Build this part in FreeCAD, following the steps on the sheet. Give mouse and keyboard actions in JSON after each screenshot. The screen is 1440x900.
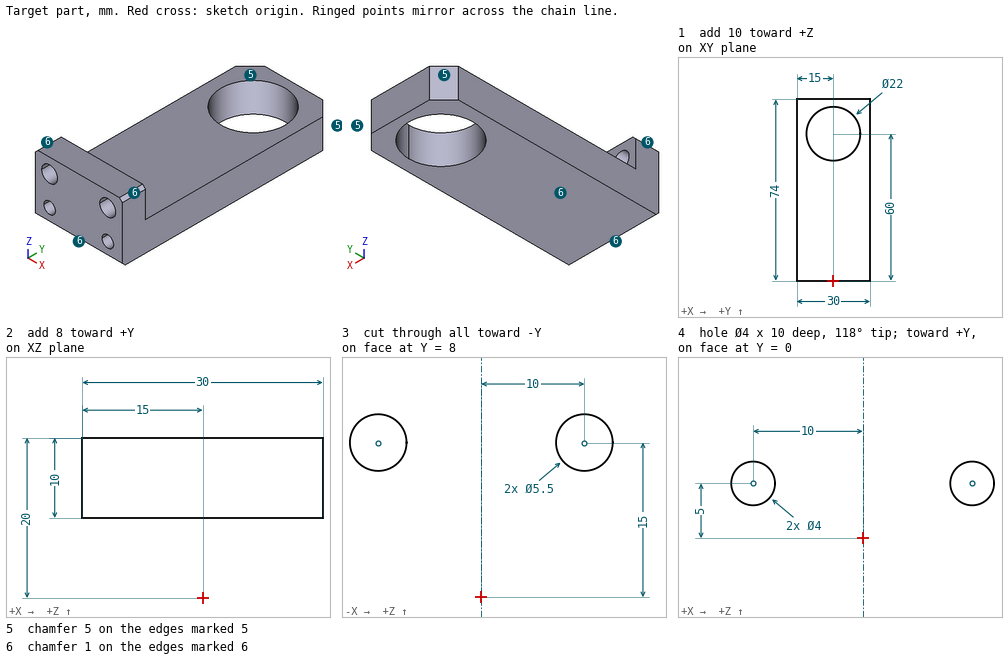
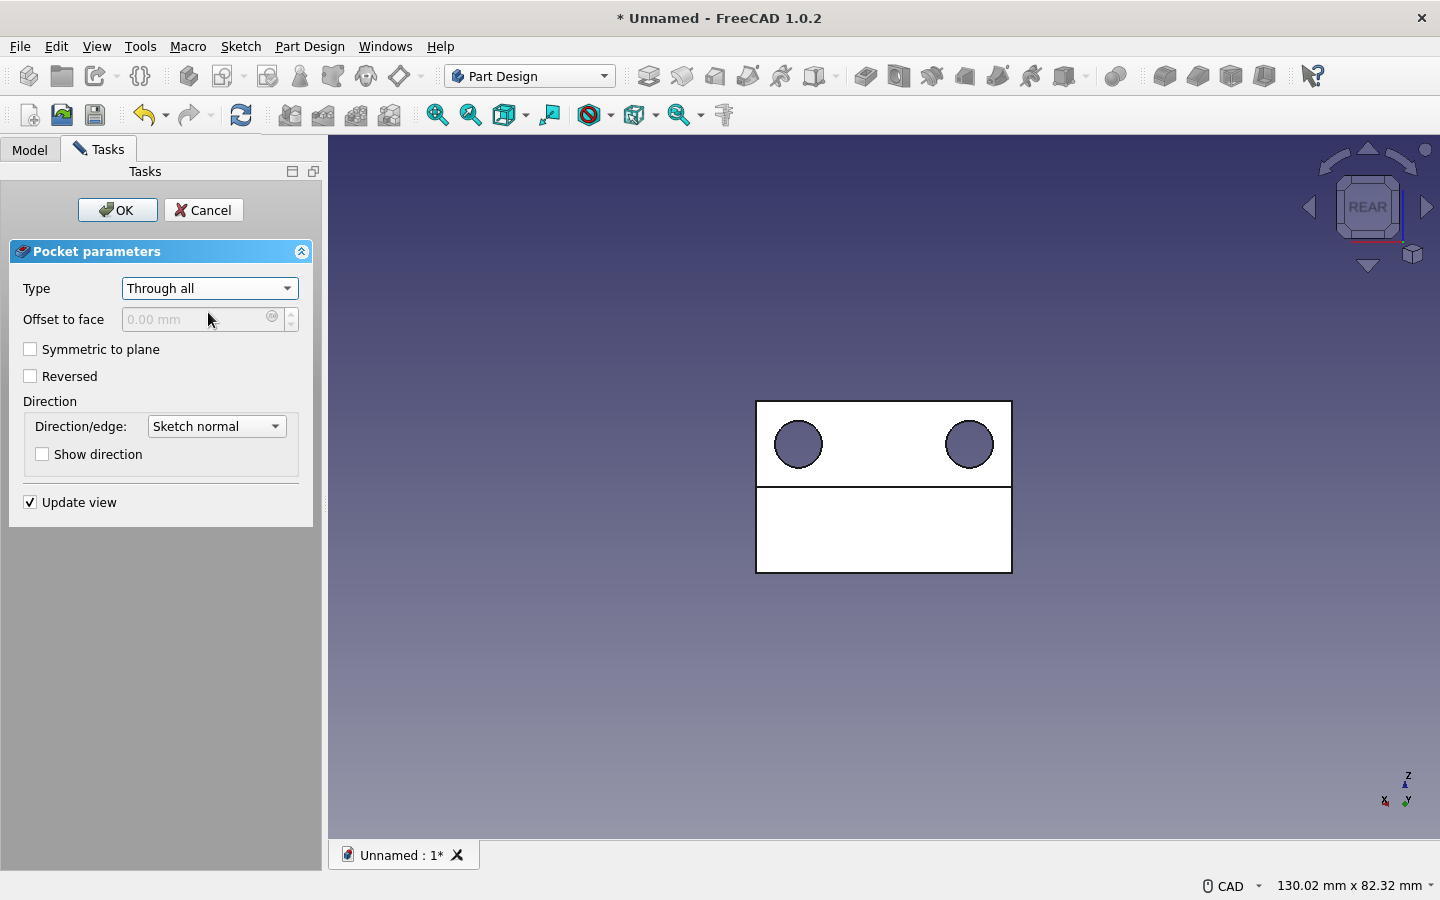
{"action": "left_click", "coordinate": [118, 210]}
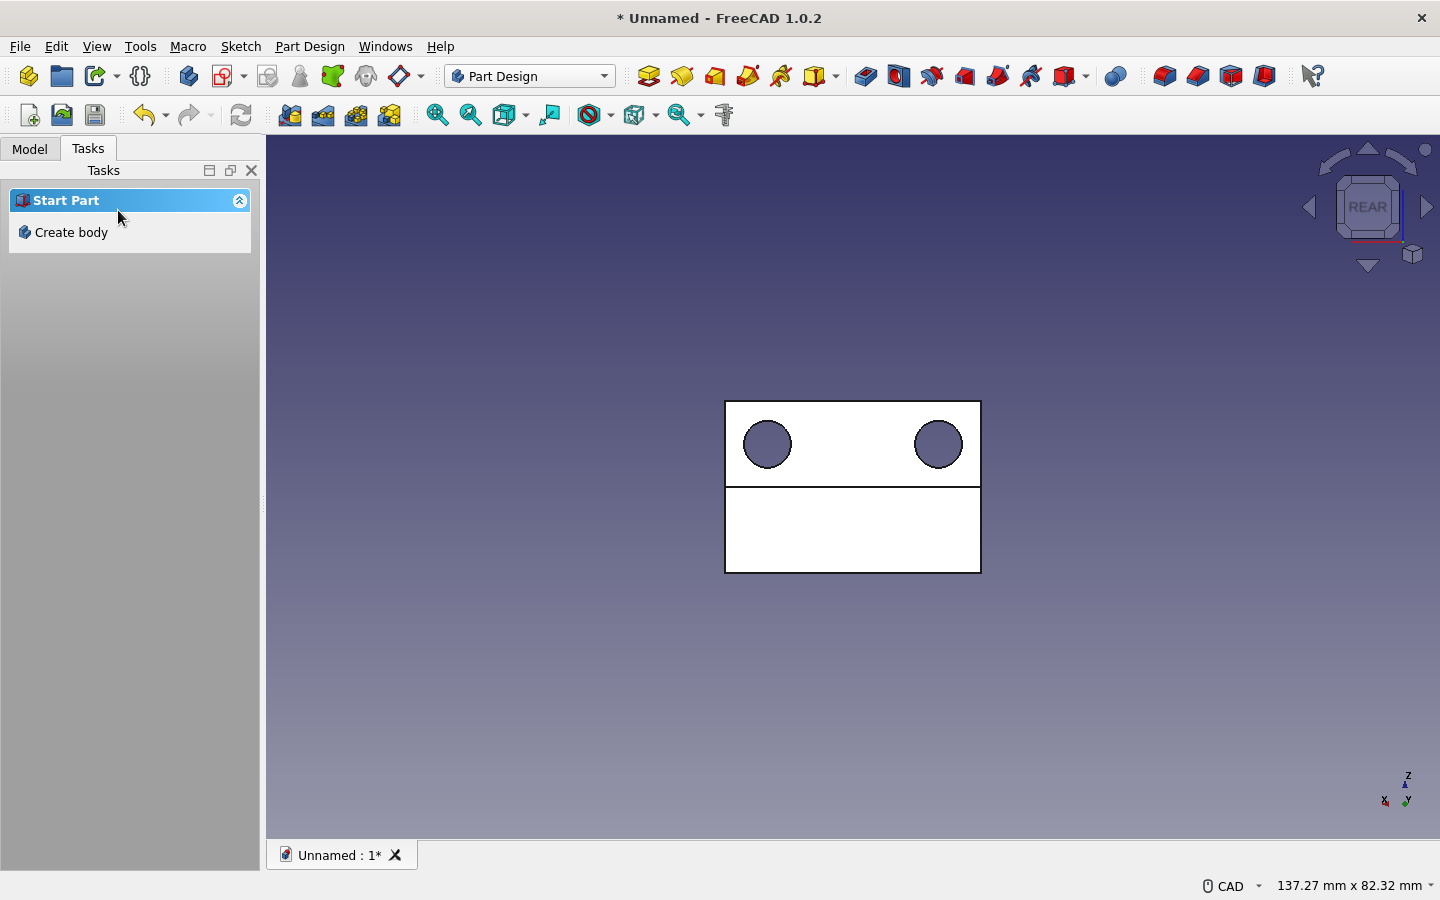
{"action": "left_click", "coordinate": [438, 116]}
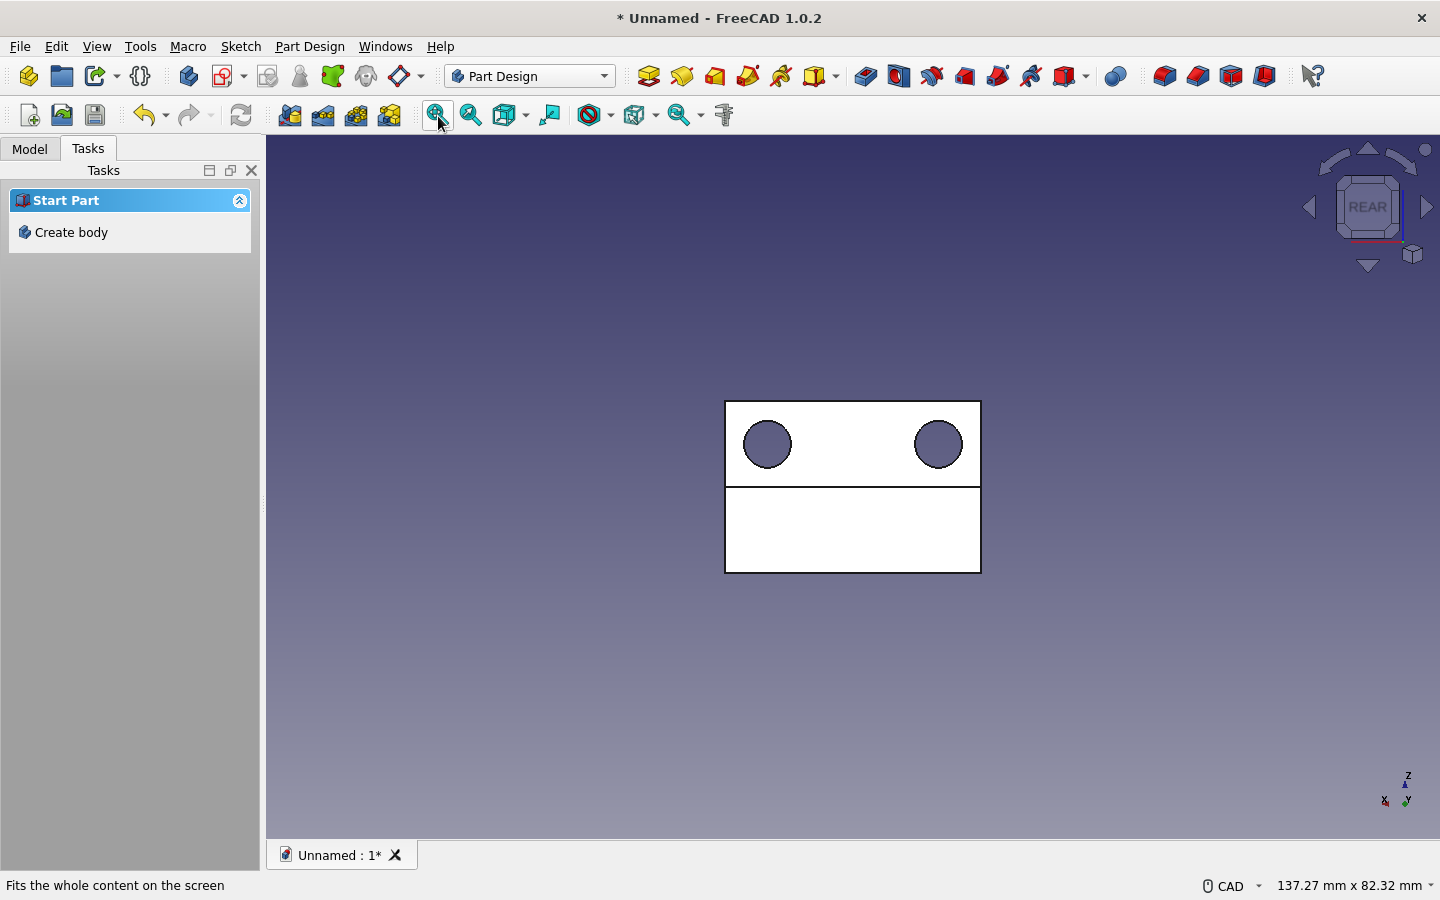
{"action": "key", "text": "0"}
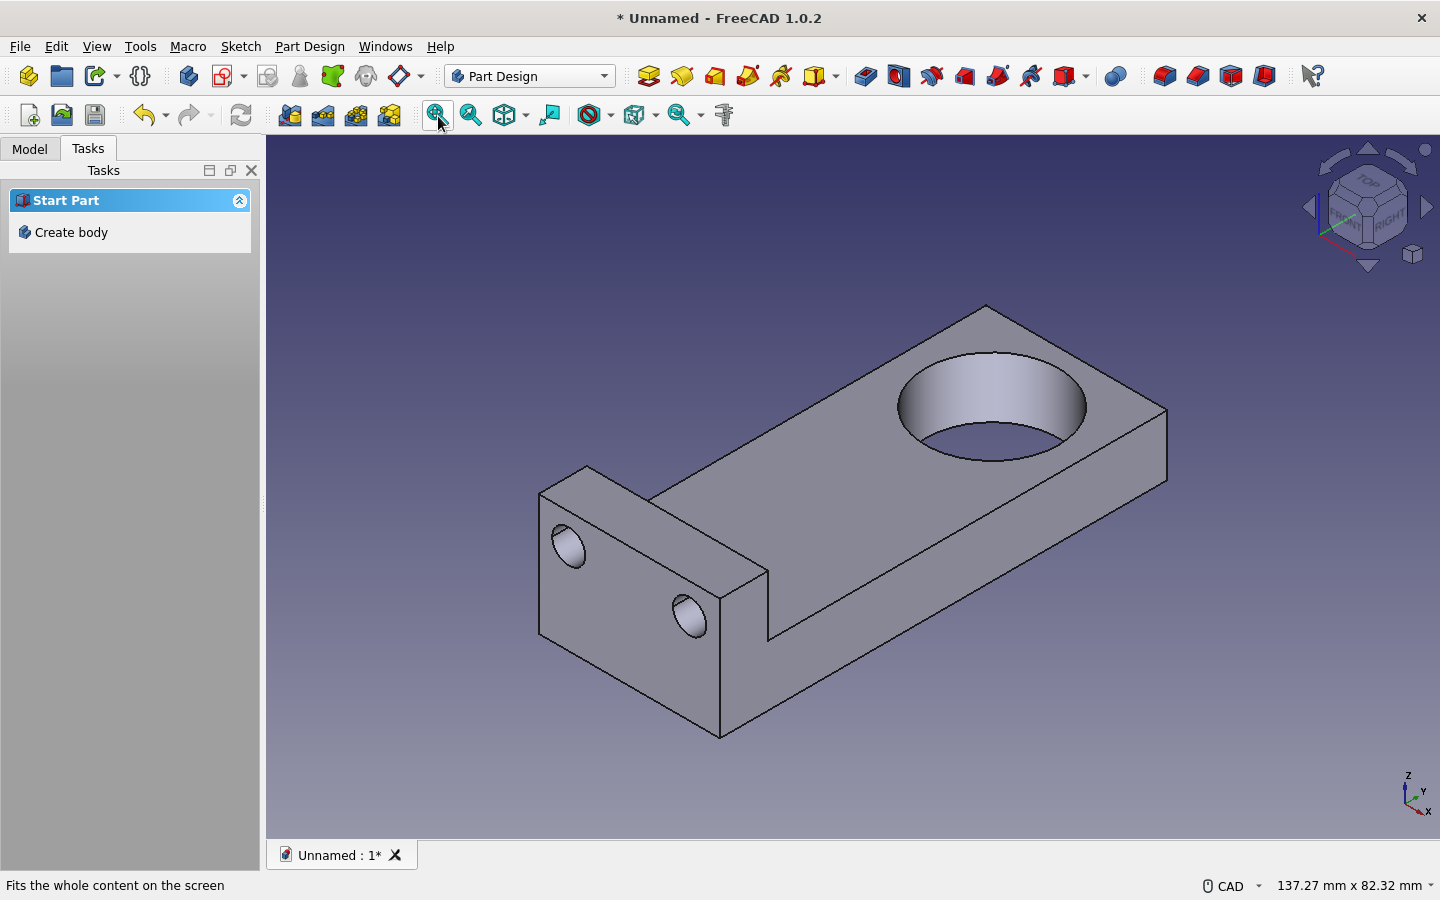
{"action": "left_click", "coordinate": [629, 615]}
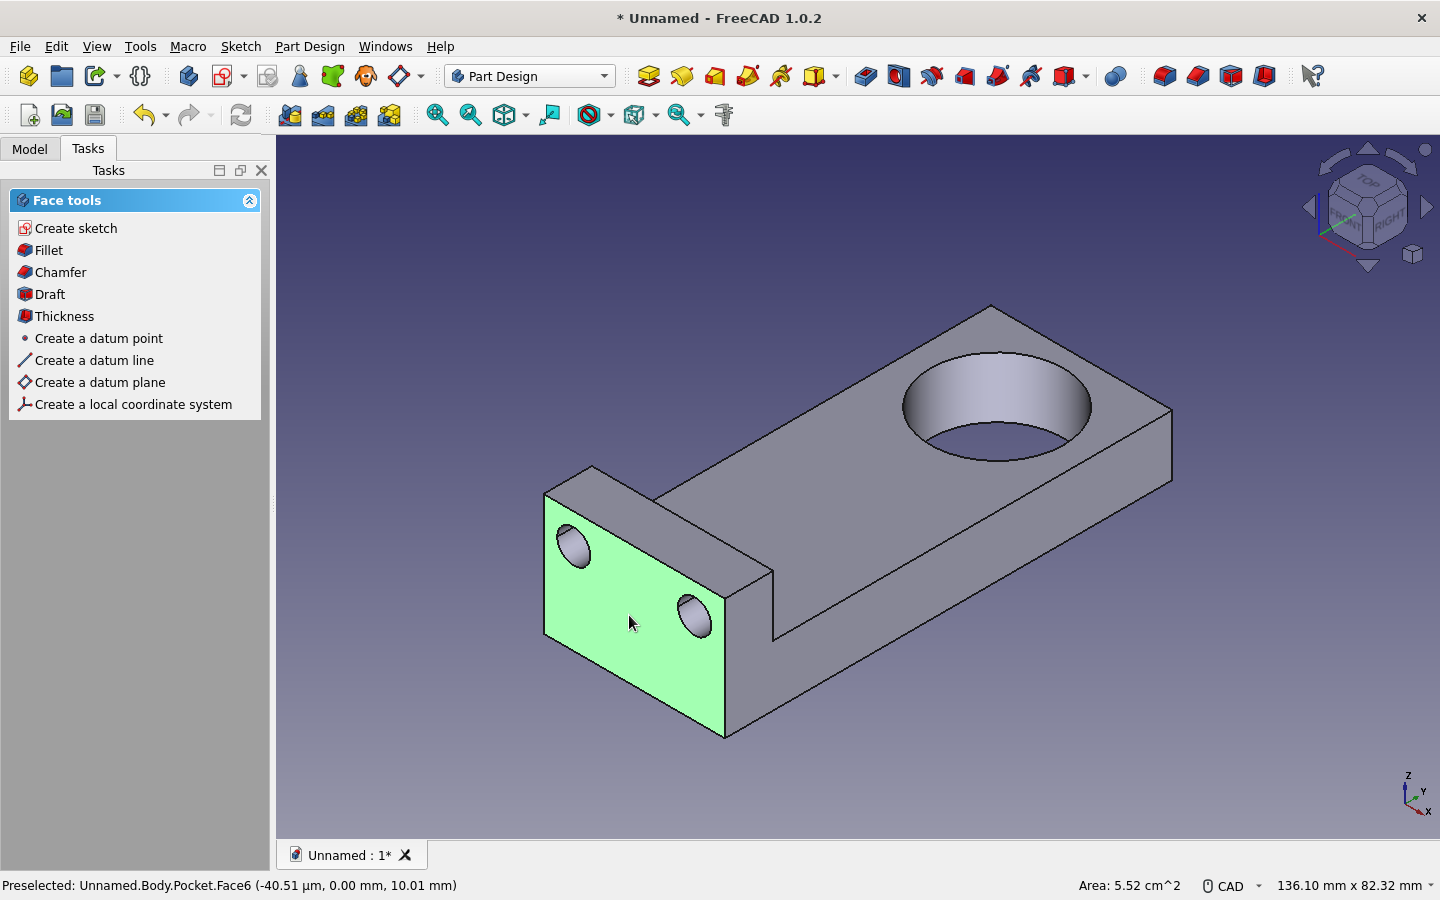
{"action": "left_click", "coordinate": [222, 76]}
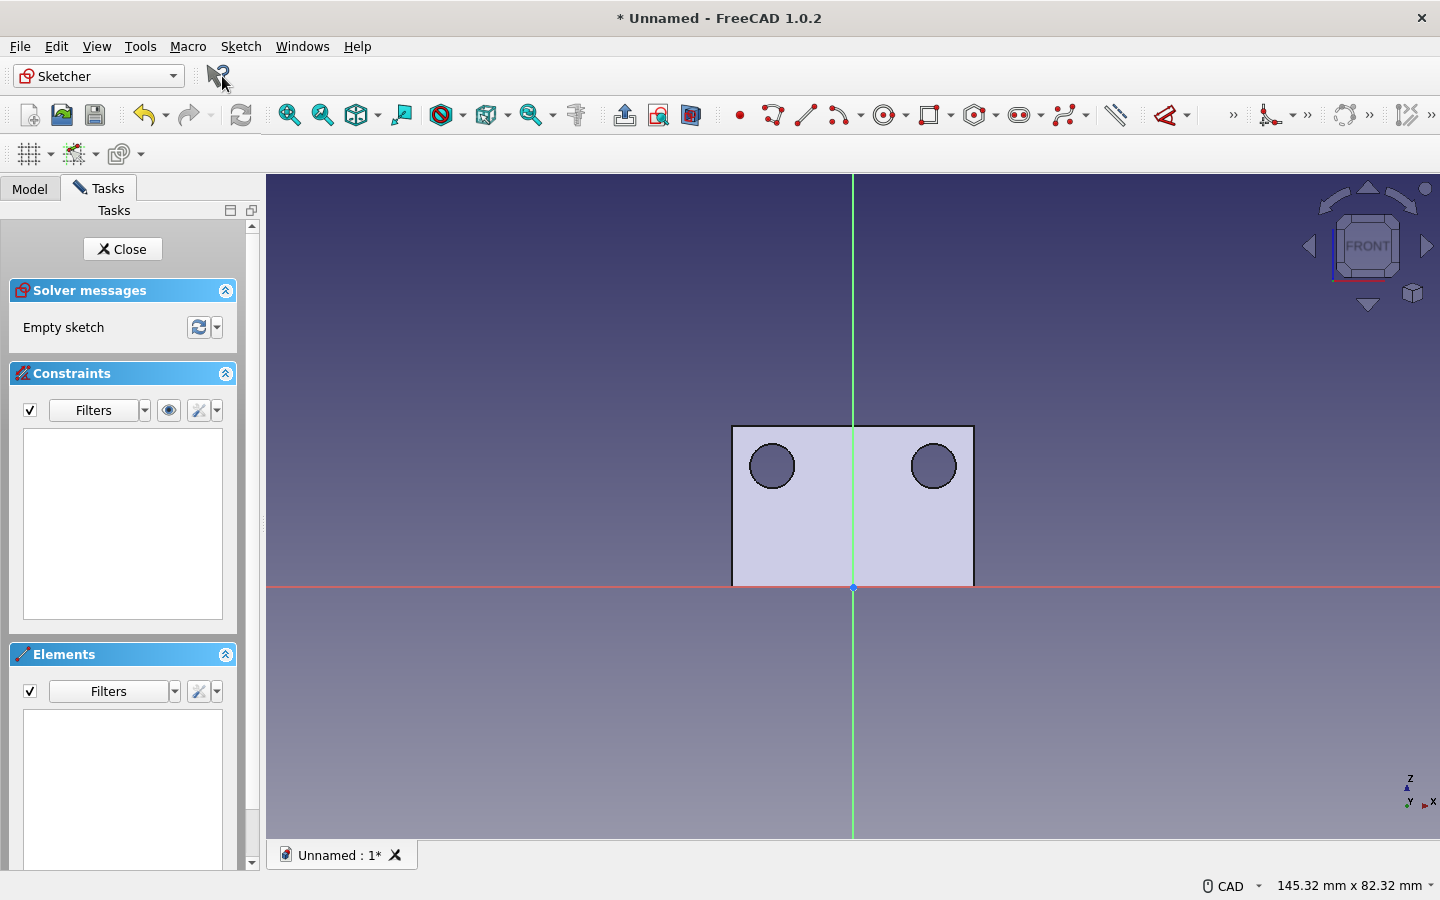
{"action": "scroll", "coordinate": [883, 582], "scroll_direction": "up", "scroll_amount": 6}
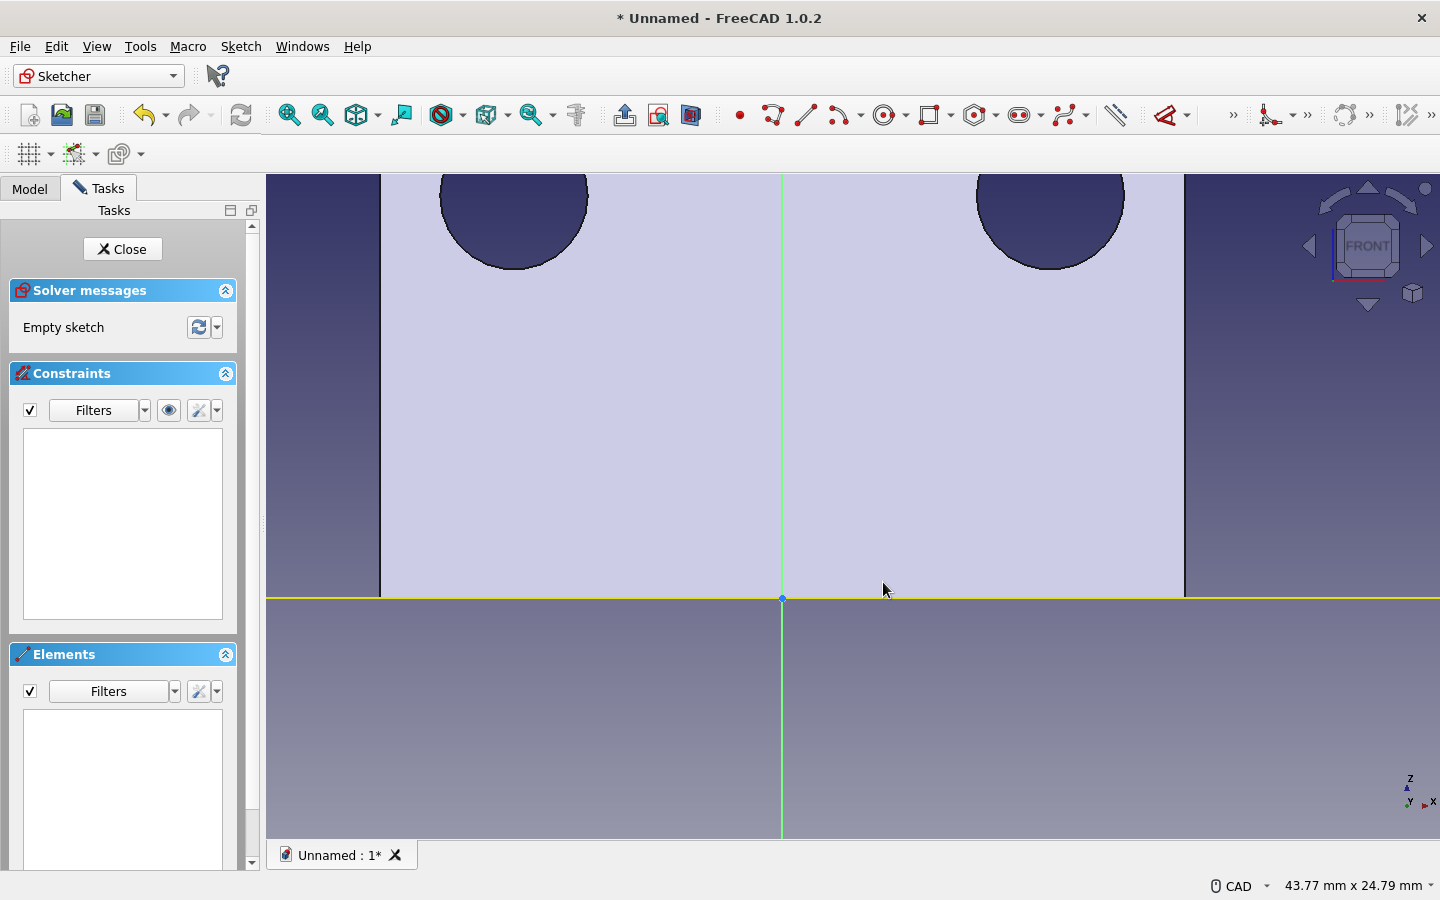
{"action": "left_click", "coordinate": [884, 116]}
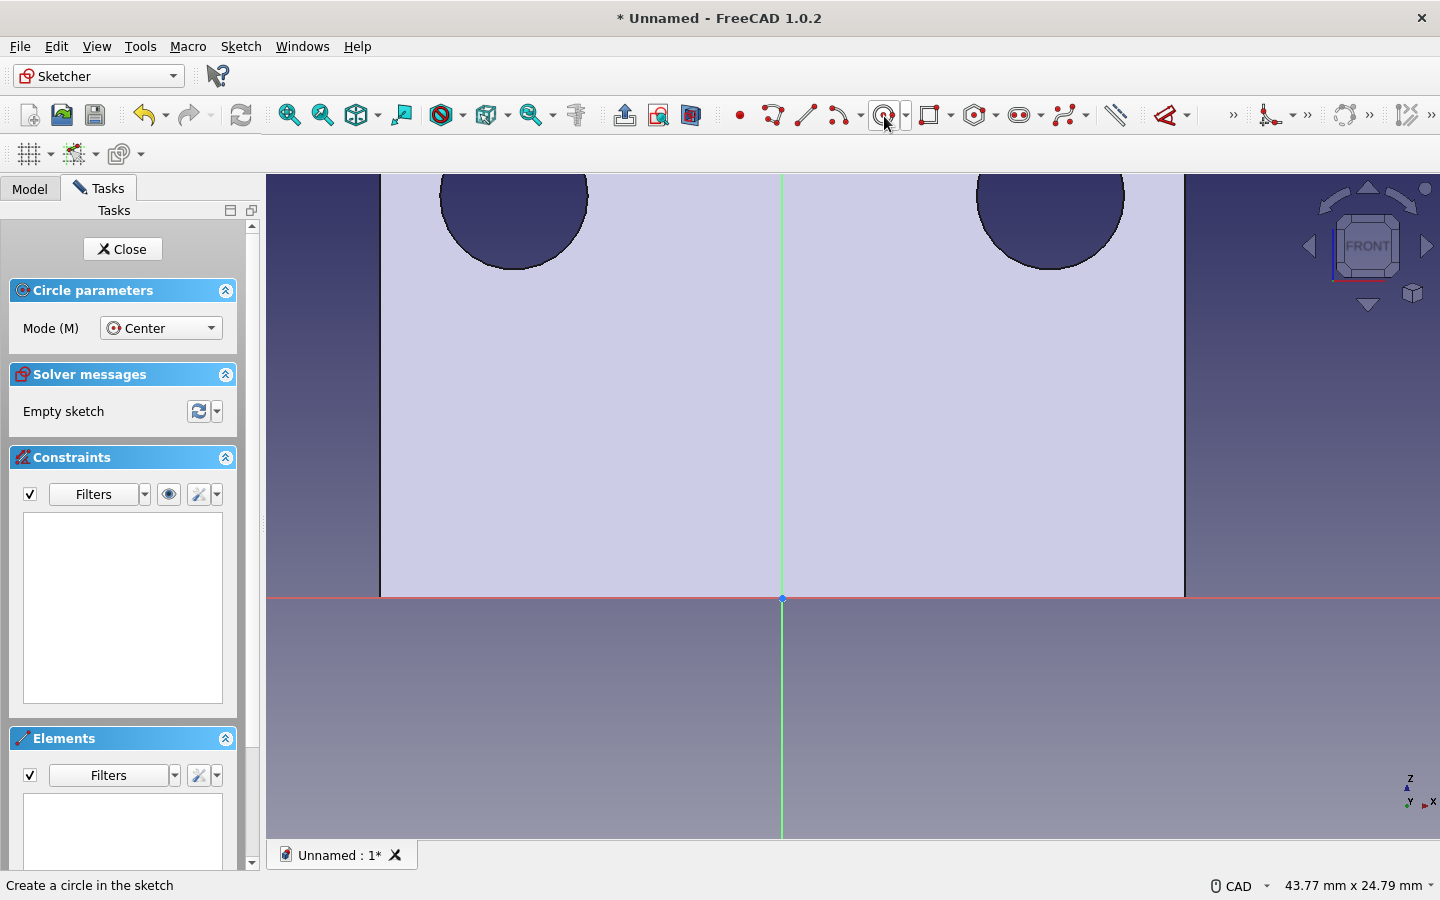
{"action": "left_click", "coordinate": [514, 464]}
{"action": "left_click", "coordinate": [552, 426]}